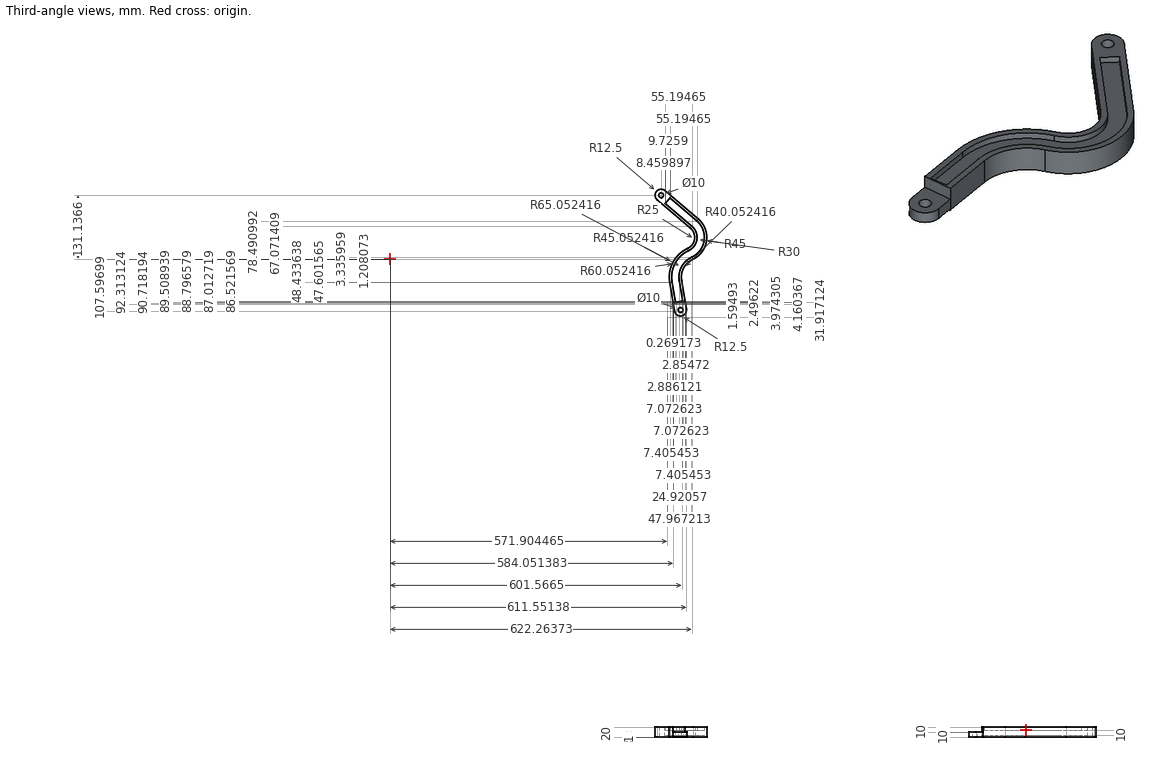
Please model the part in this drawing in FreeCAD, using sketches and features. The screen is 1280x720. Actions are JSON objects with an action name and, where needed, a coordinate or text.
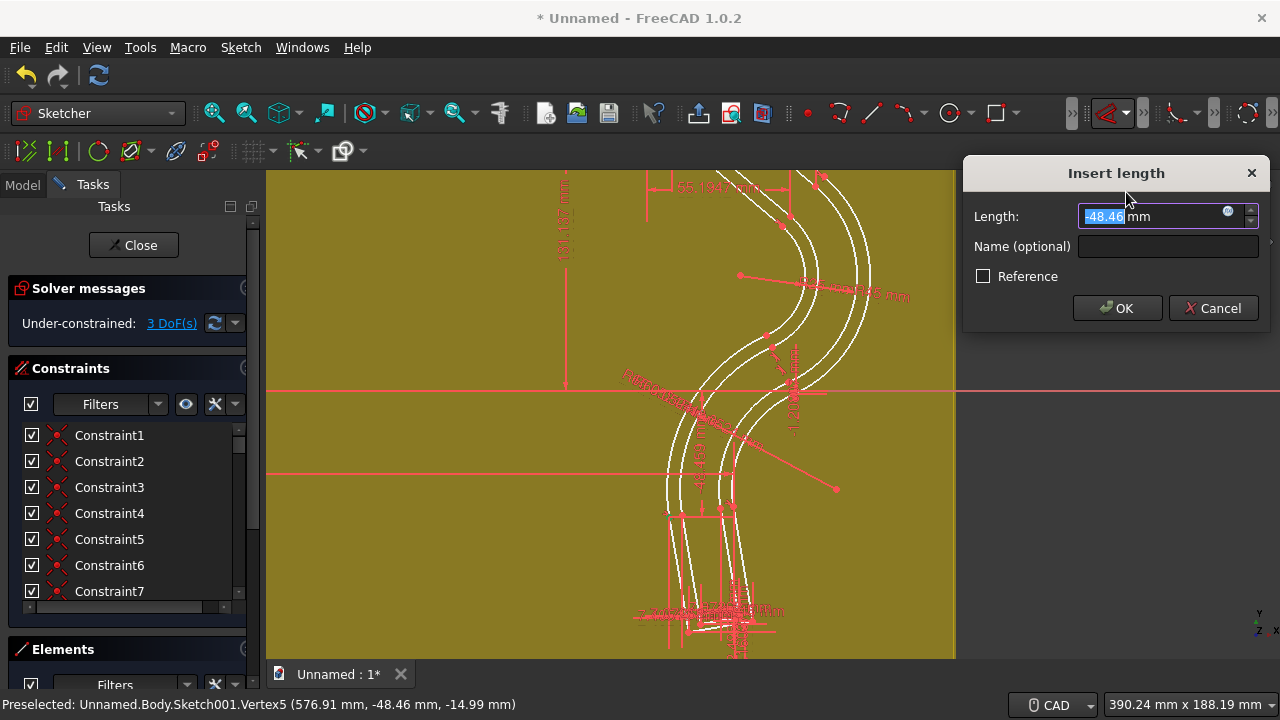
{"action": "type", "text": "-48.433638"}
{"action": "key", "text": "Return"}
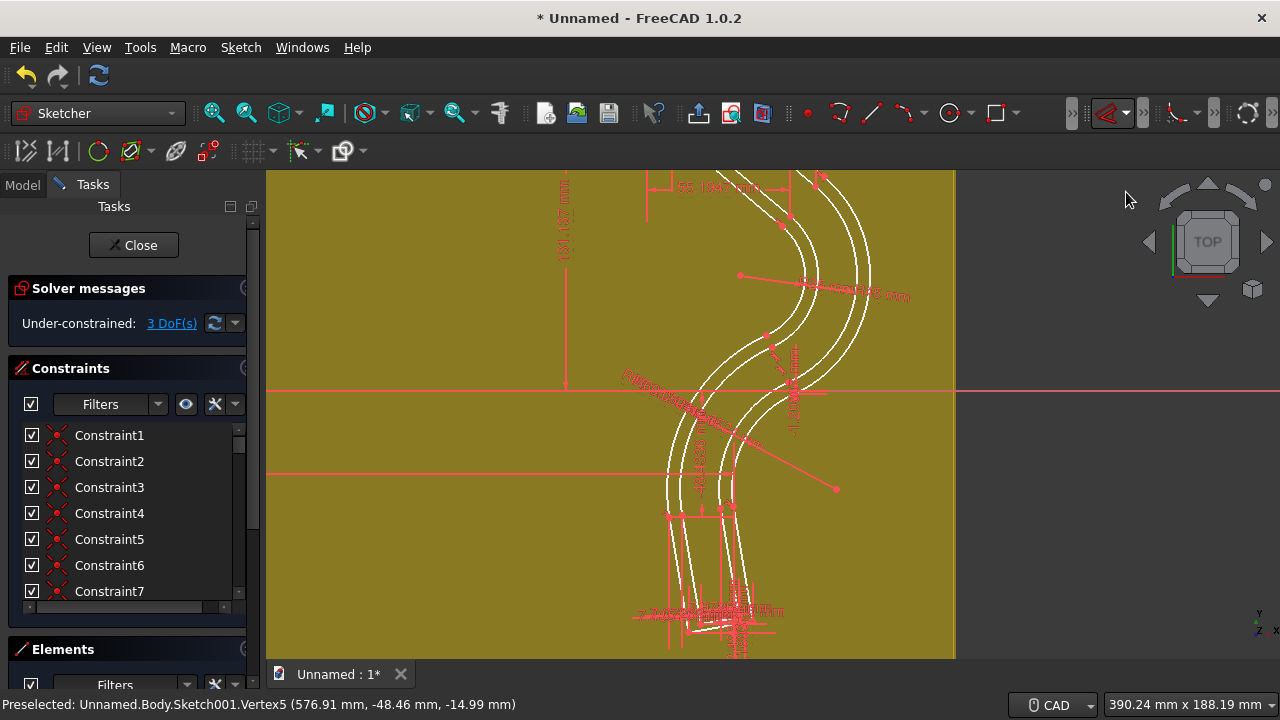
{"action": "scroll", "coordinate": [670, 519], "scroll_direction": "down", "scroll_amount": 3}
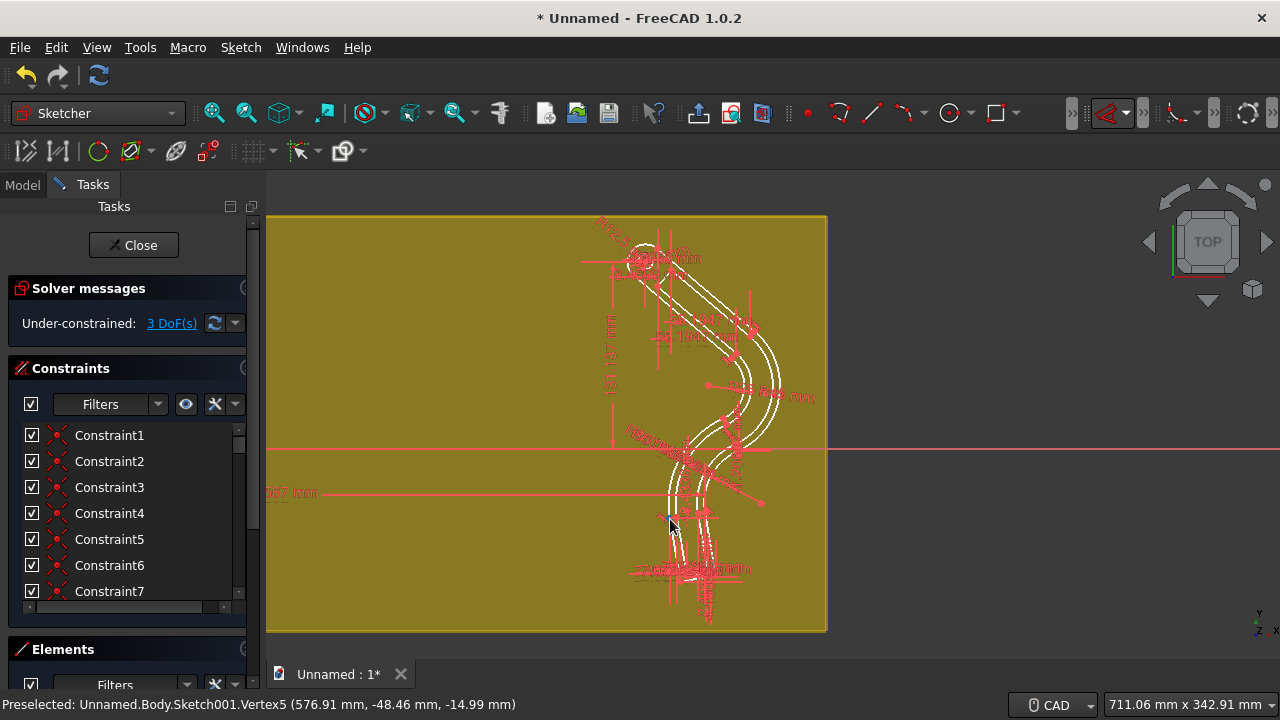
{"action": "scroll", "coordinate": [680, 582], "scroll_direction": "up", "scroll_amount": 3}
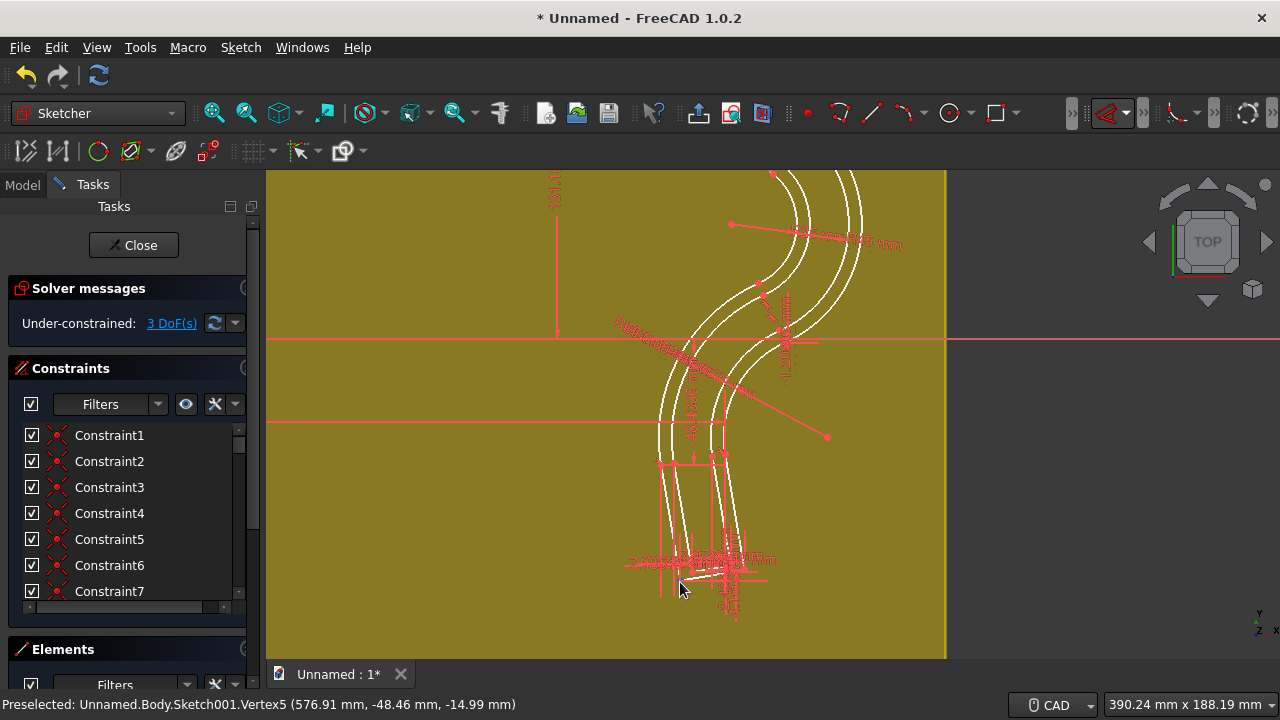
{"action": "left_click", "coordinate": [680, 581]}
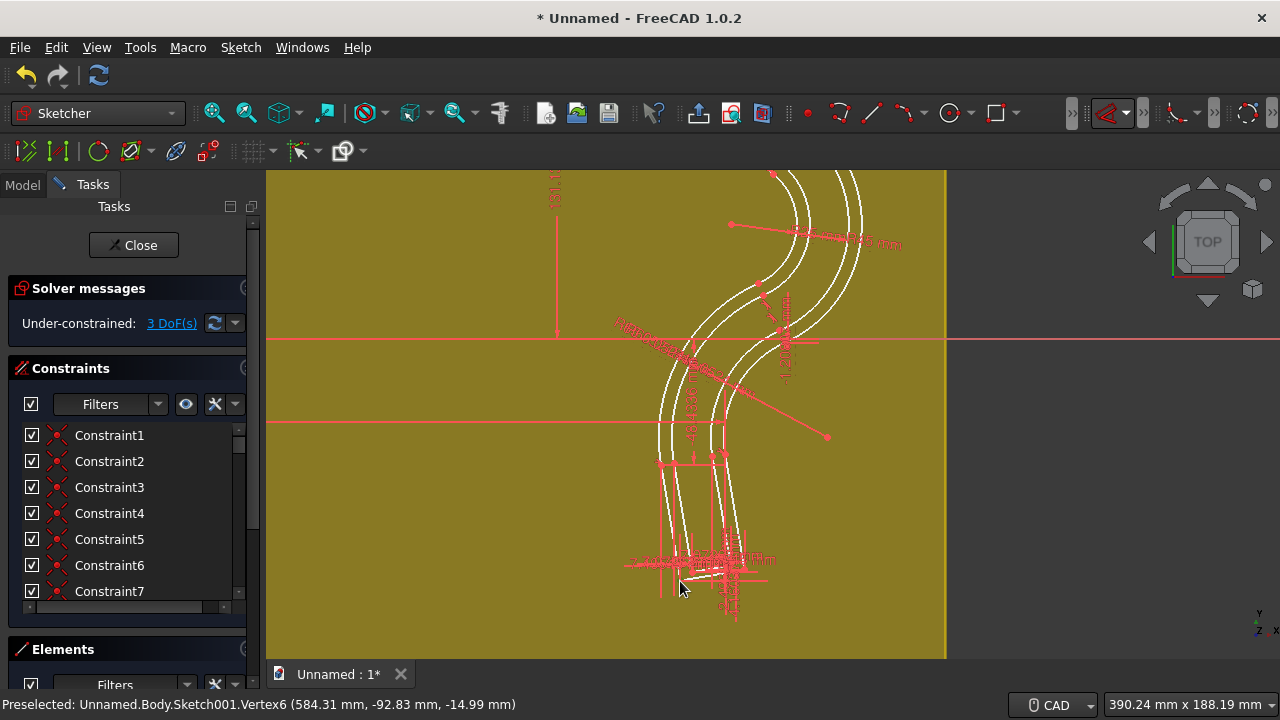
{"action": "key", "text": "i"}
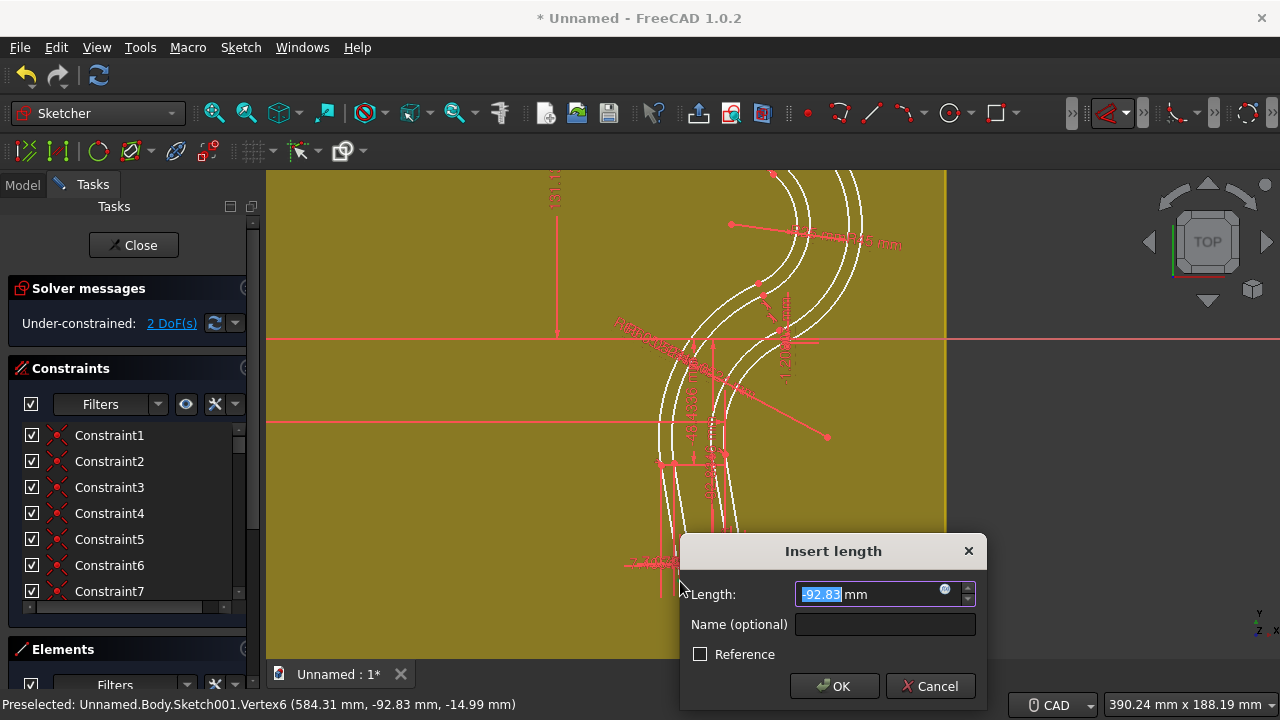
{"action": "type", "text": "-92.313124"}
{"action": "key", "text": "Return"}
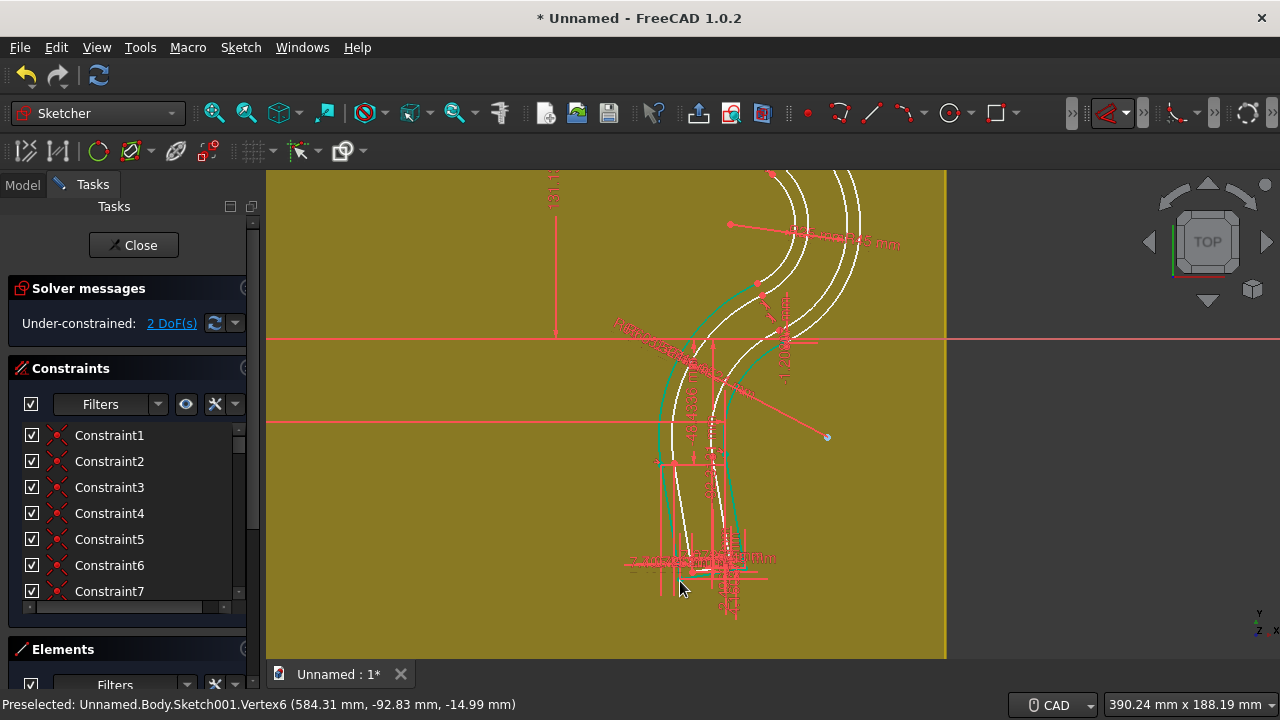
{"action": "left_click", "coordinate": [731, 566]}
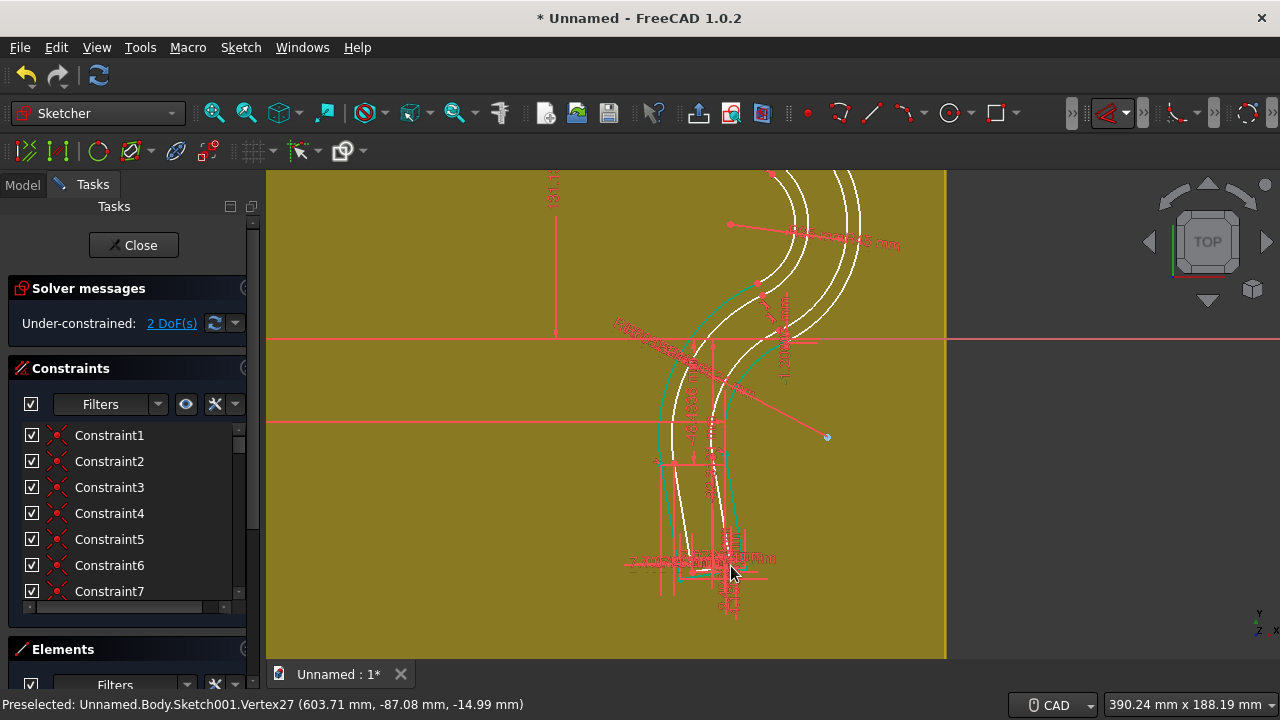
{"action": "key", "text": "i"}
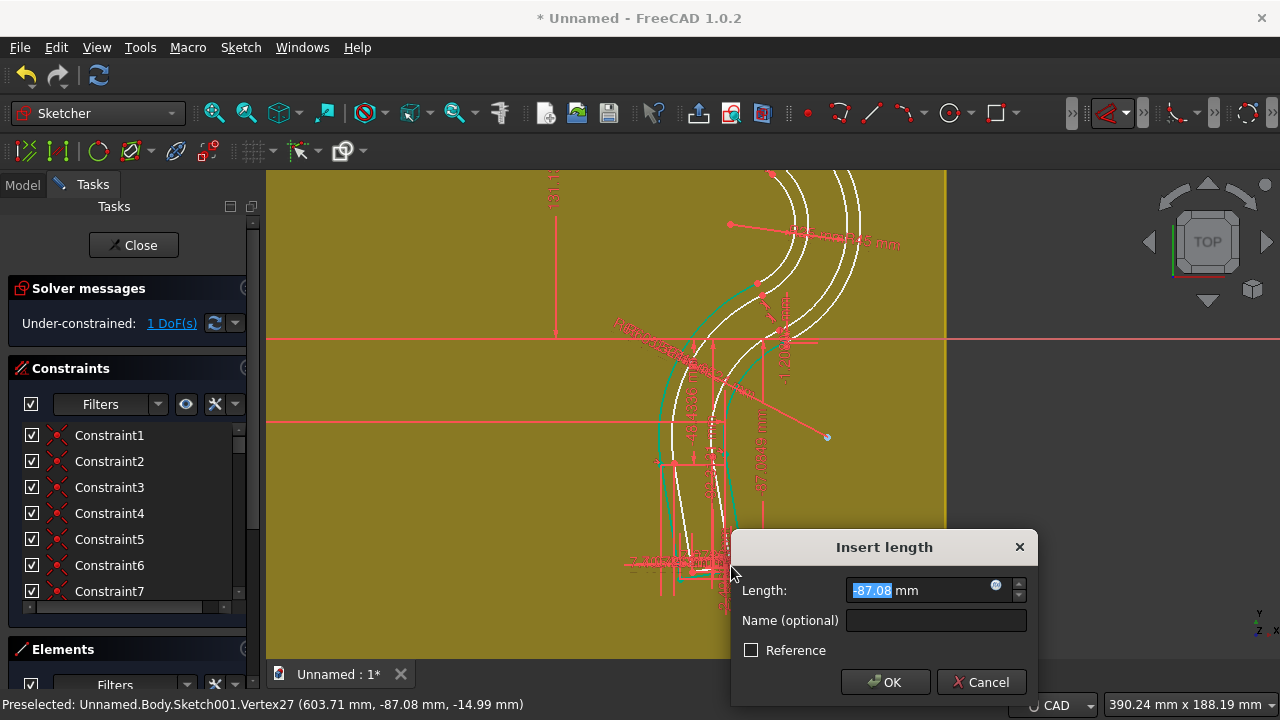
{"action": "type", "text": "-87.012719"}
{"action": "key", "text": "Return"}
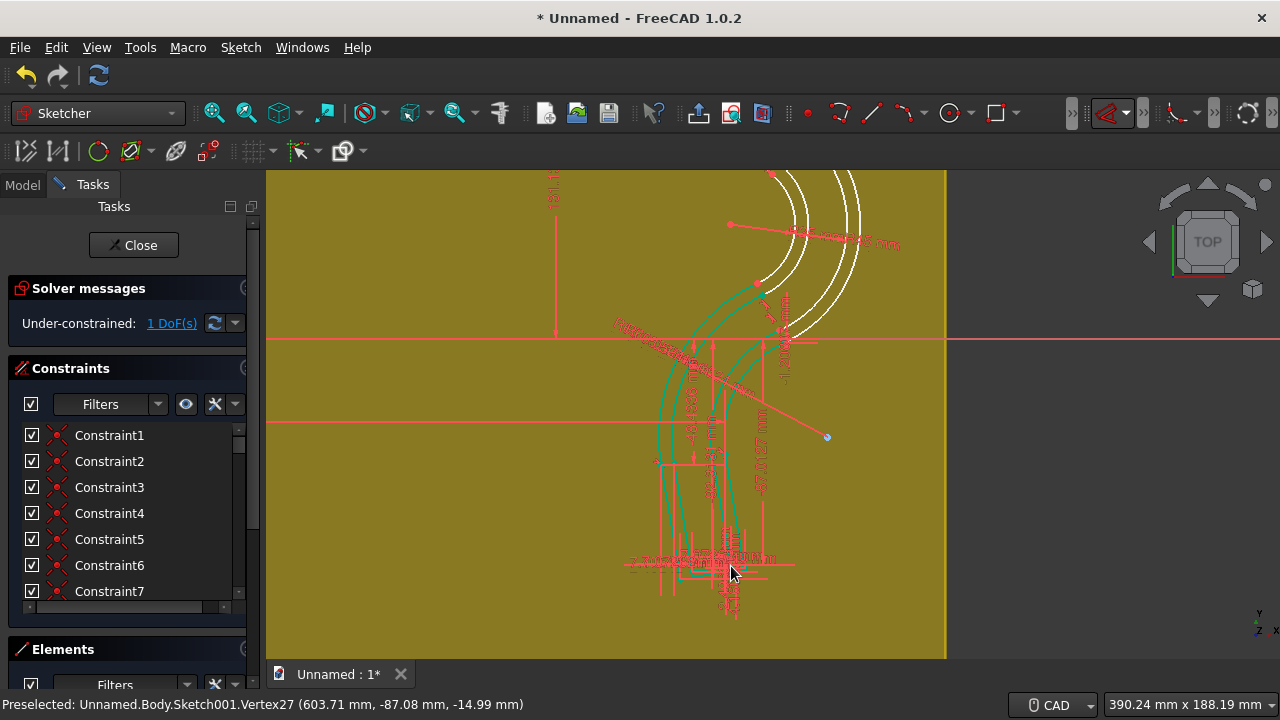
{"action": "scroll", "coordinate": [680, 582], "scroll_direction": "down", "scroll_amount": 3}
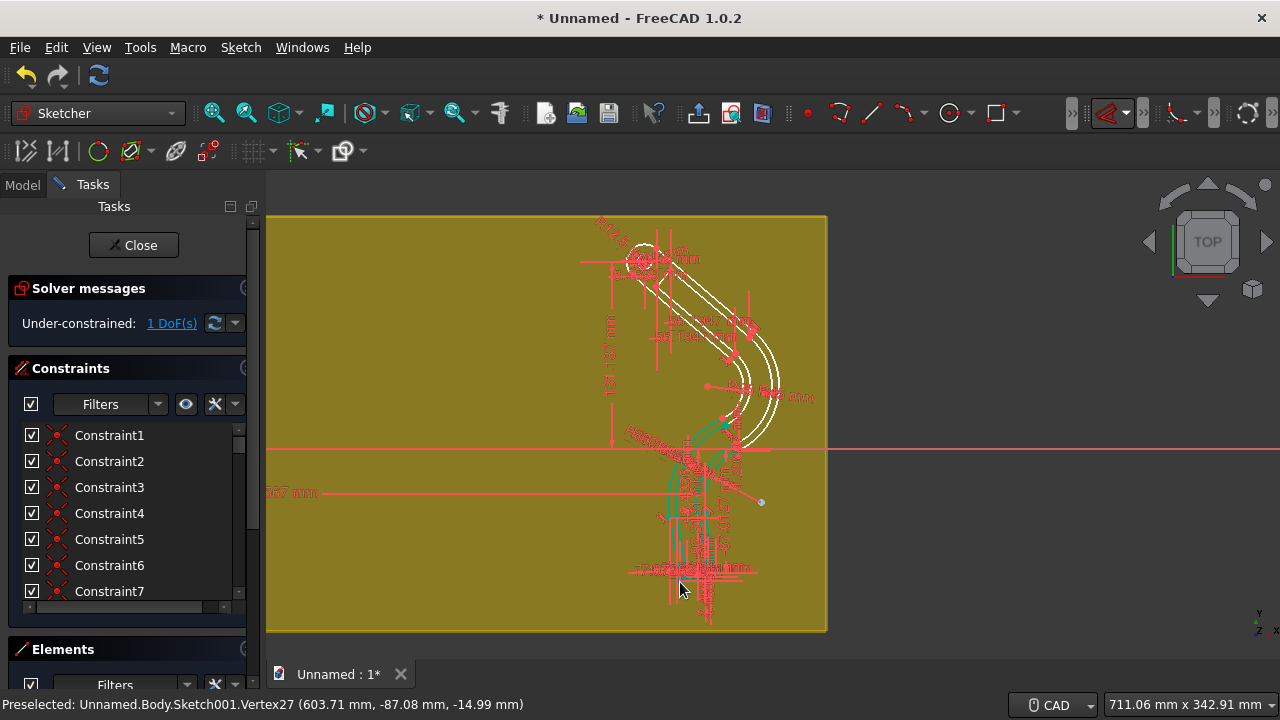
{"action": "scroll", "coordinate": [735, 354], "scroll_direction": "up", "scroll_amount": 3}